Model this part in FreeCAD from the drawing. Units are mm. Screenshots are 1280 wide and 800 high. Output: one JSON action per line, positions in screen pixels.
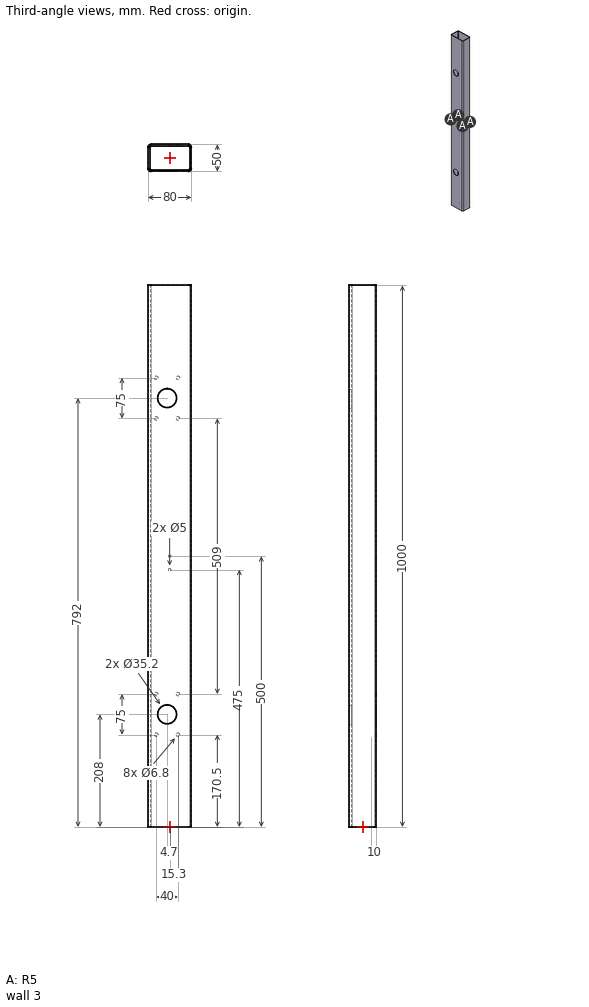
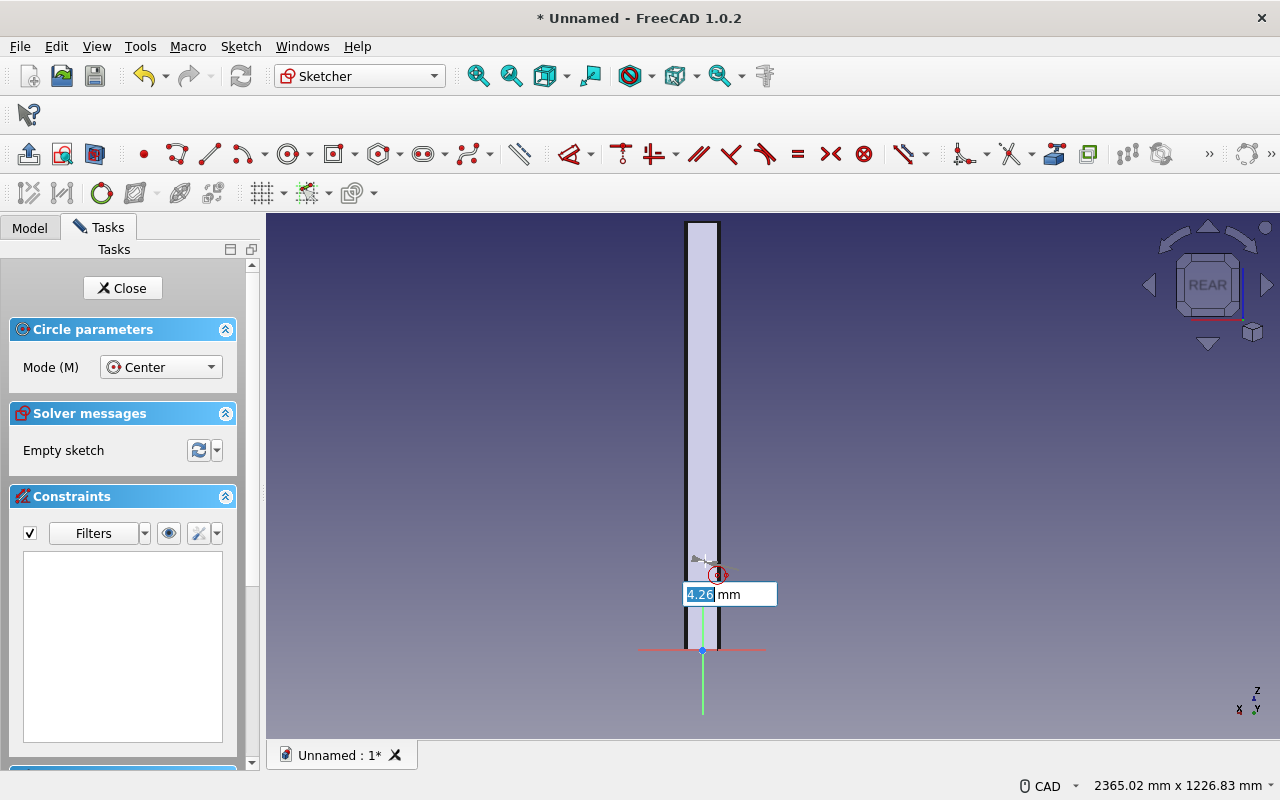
{"action": "scroll", "coordinate": [710, 556], "scroll_direction": "up", "scroll_amount": 4}
{"action": "mouse_move", "coordinate": [709, 555]}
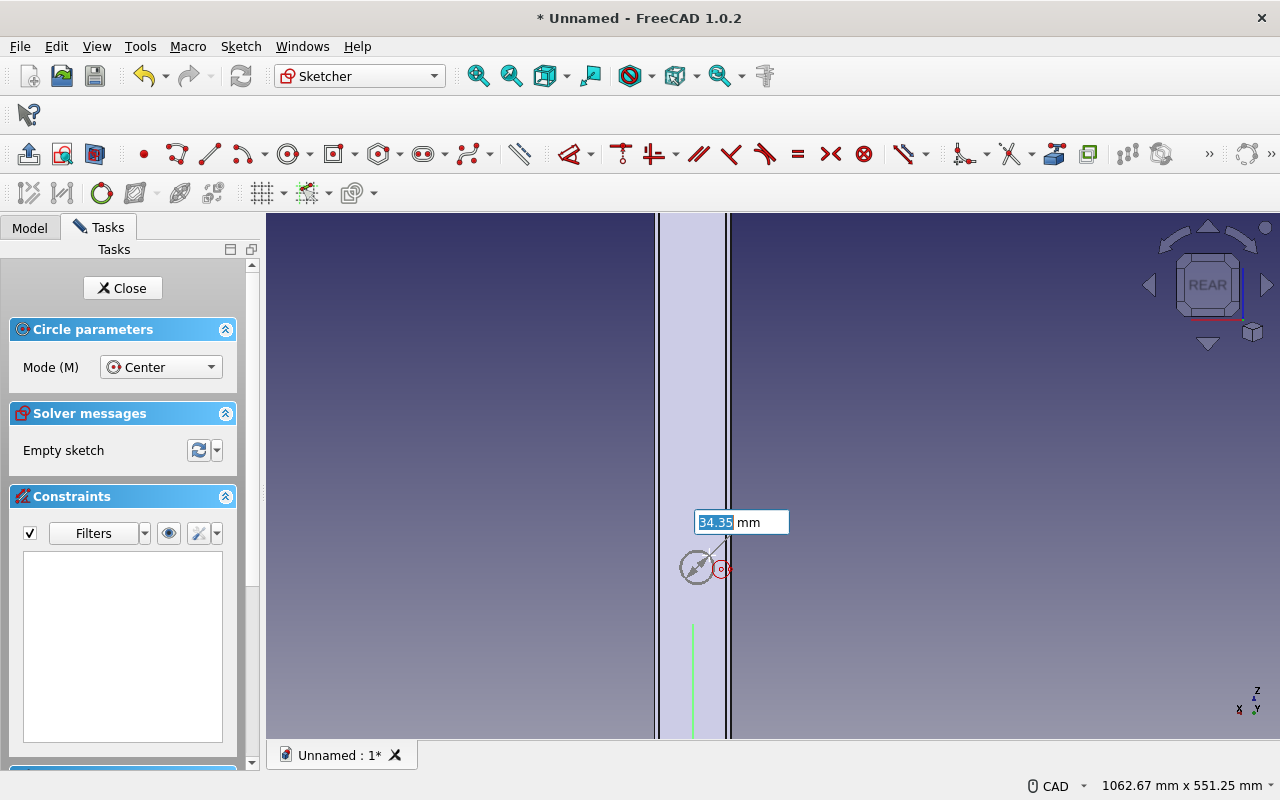
{"action": "type", "text": "35.2"}
{"action": "key", "text": "Return"}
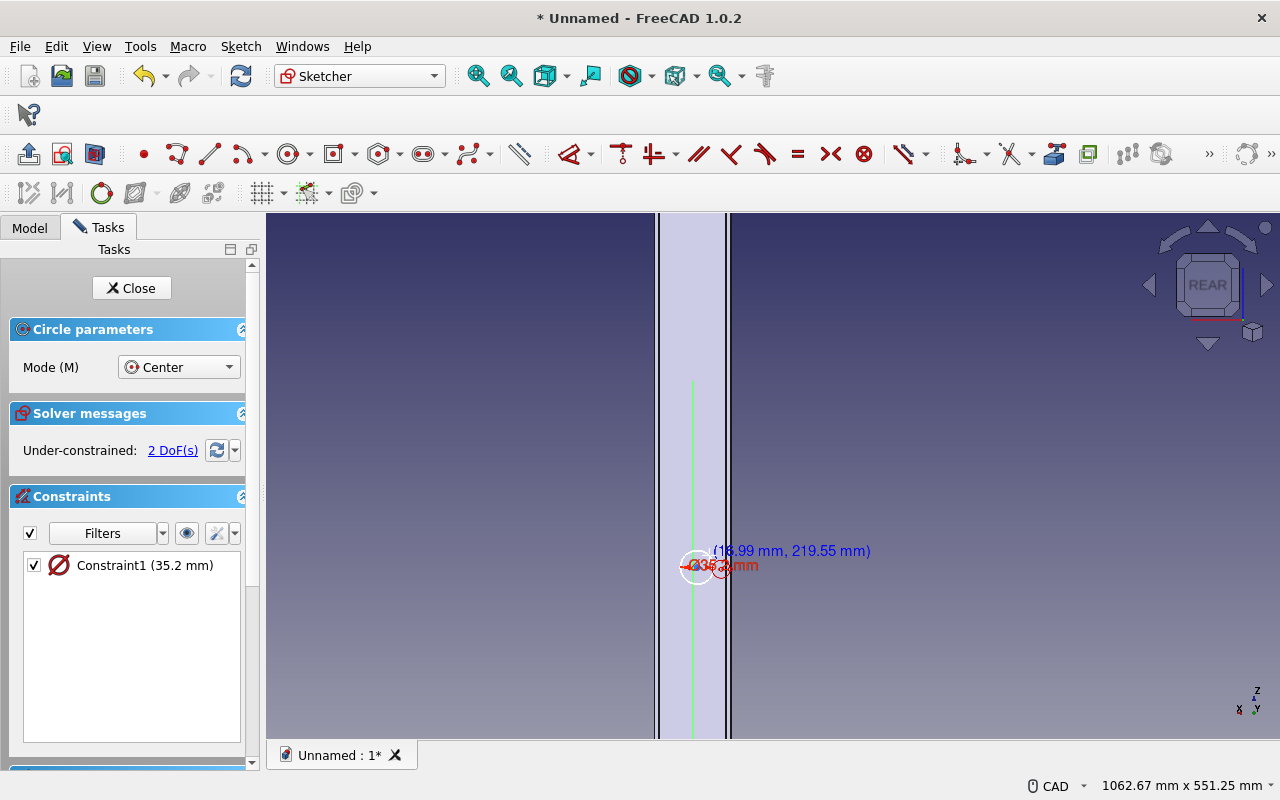
{"action": "scroll", "coordinate": [710, 555], "scroll_direction": "down", "scroll_amount": 4}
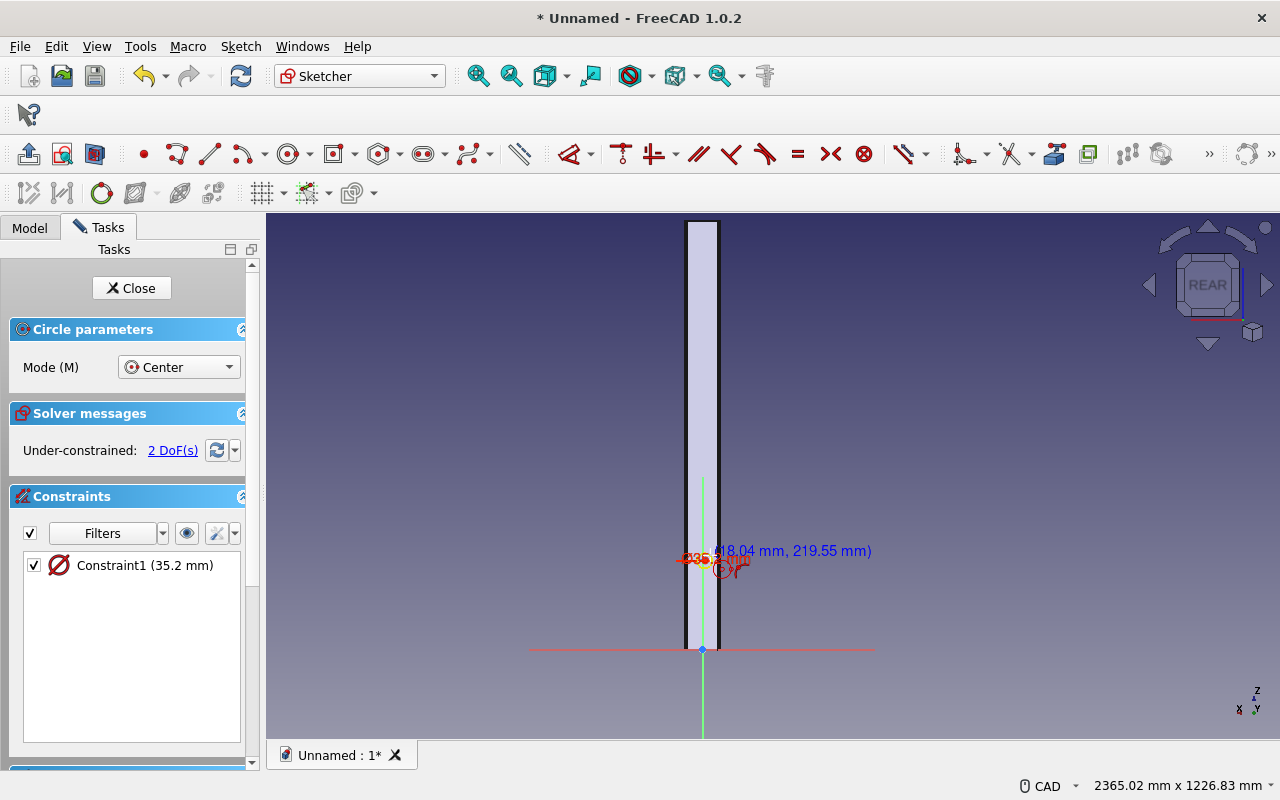
{"action": "scroll", "coordinate": [705, 310], "scroll_direction": "up", "scroll_amount": 11}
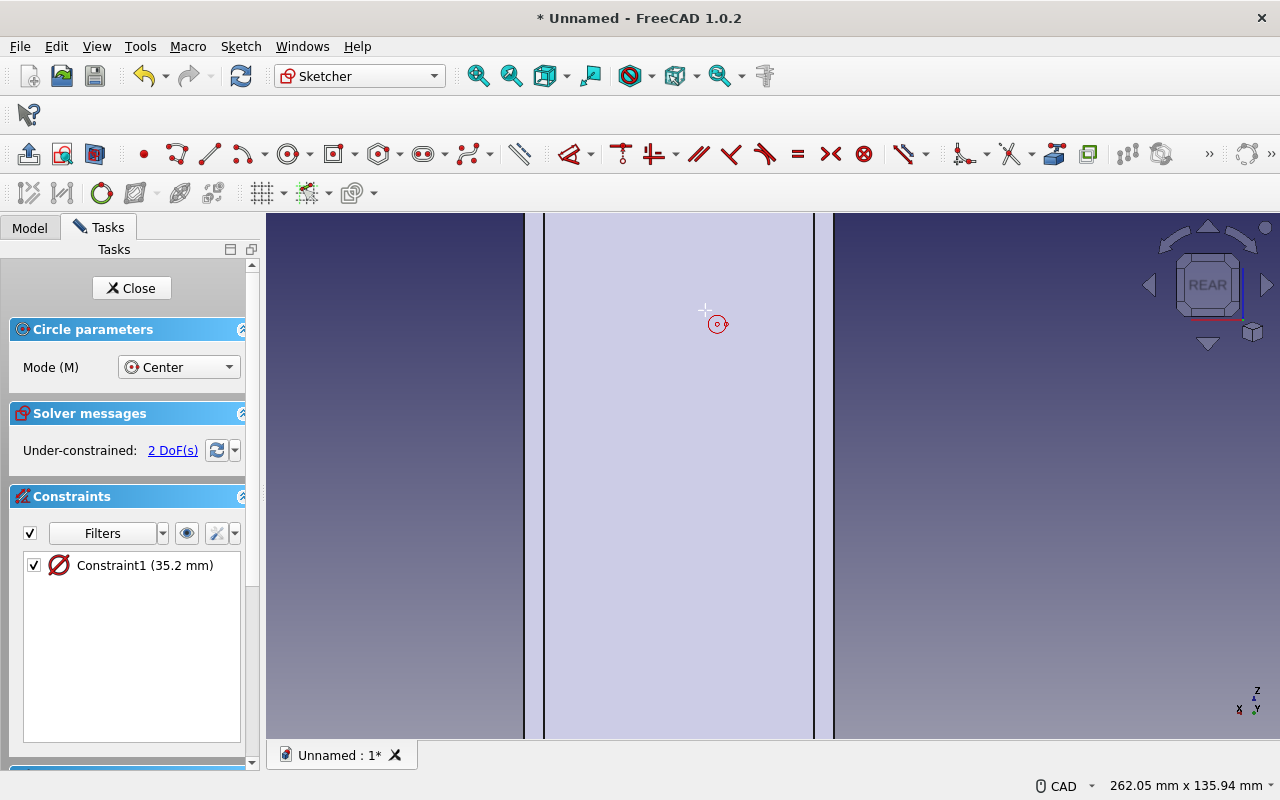
{"action": "left_click", "coordinate": [697, 312]}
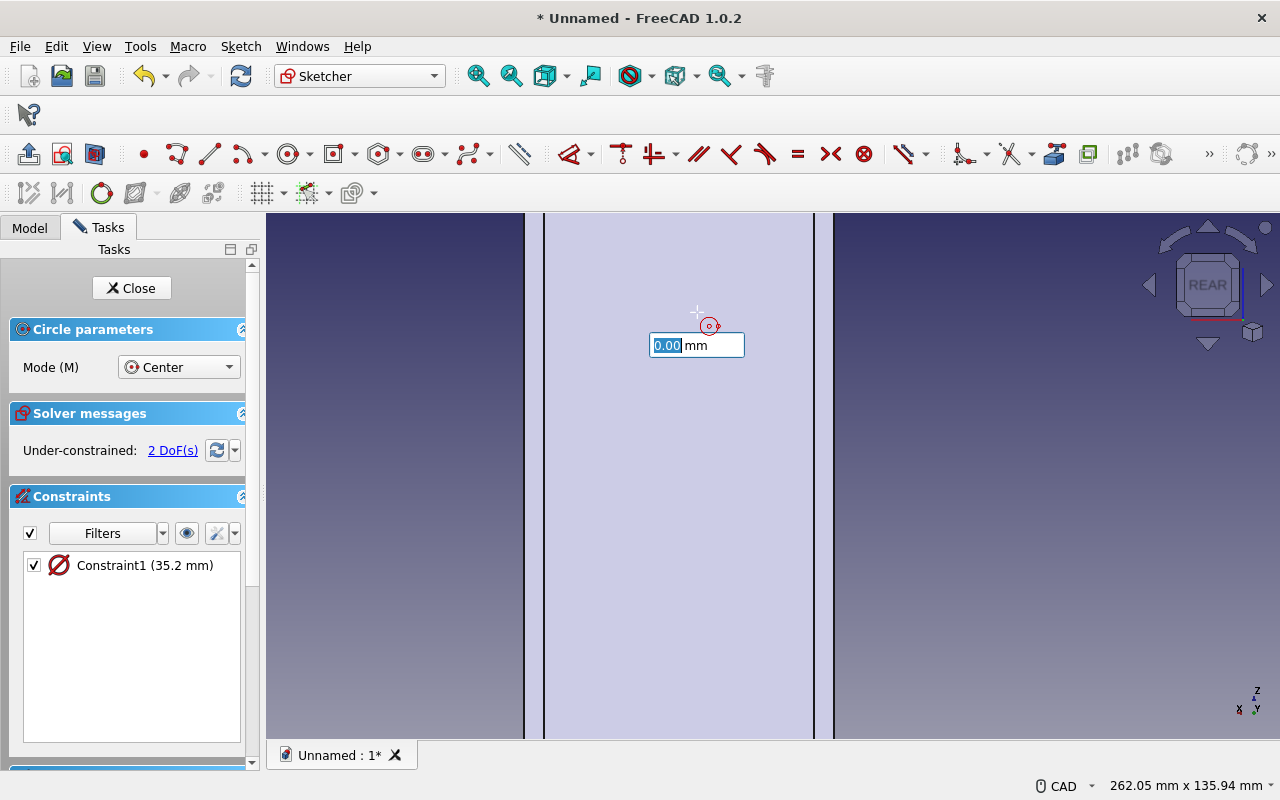
{"action": "scroll", "coordinate": [705, 310], "scroll_direction": "down", "scroll_amount": 11}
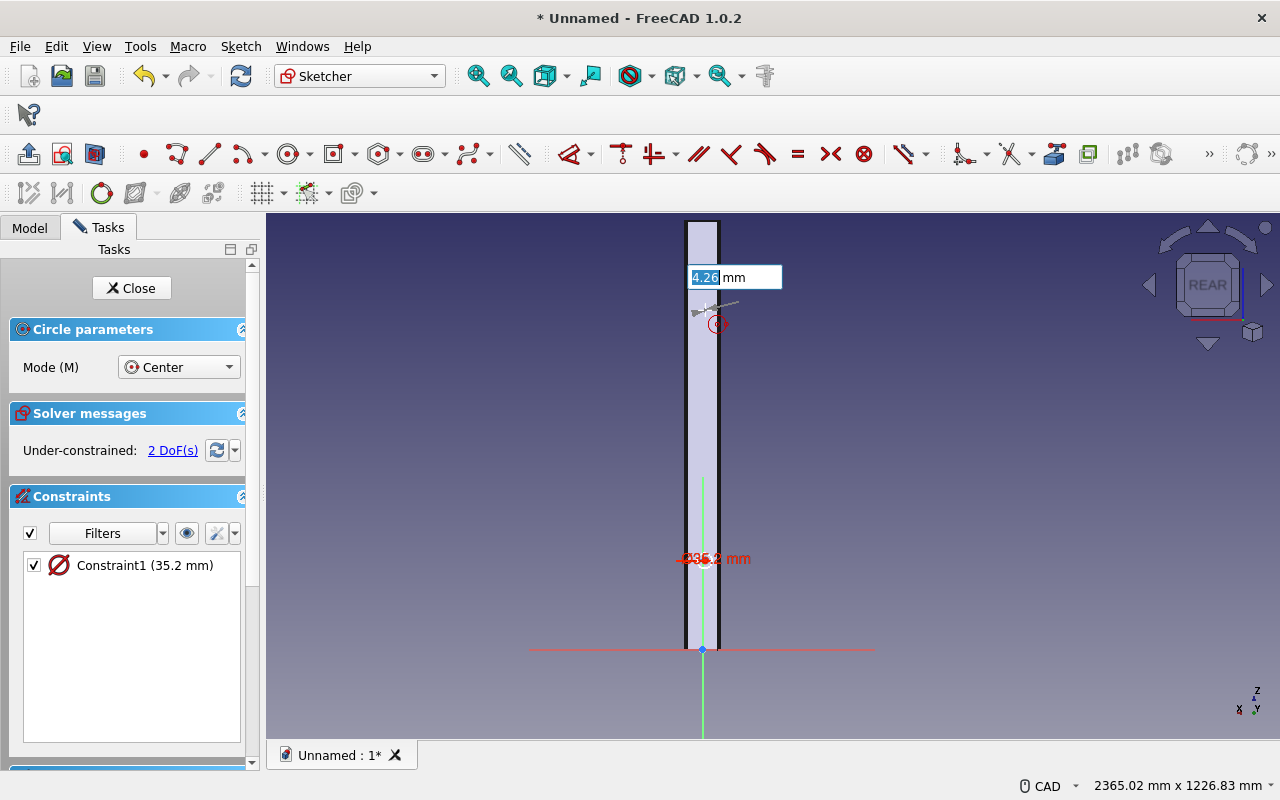
{"action": "scroll", "coordinate": [710, 305], "scroll_direction": "up", "scroll_amount": 4}
{"action": "mouse_move", "coordinate": [709, 305]}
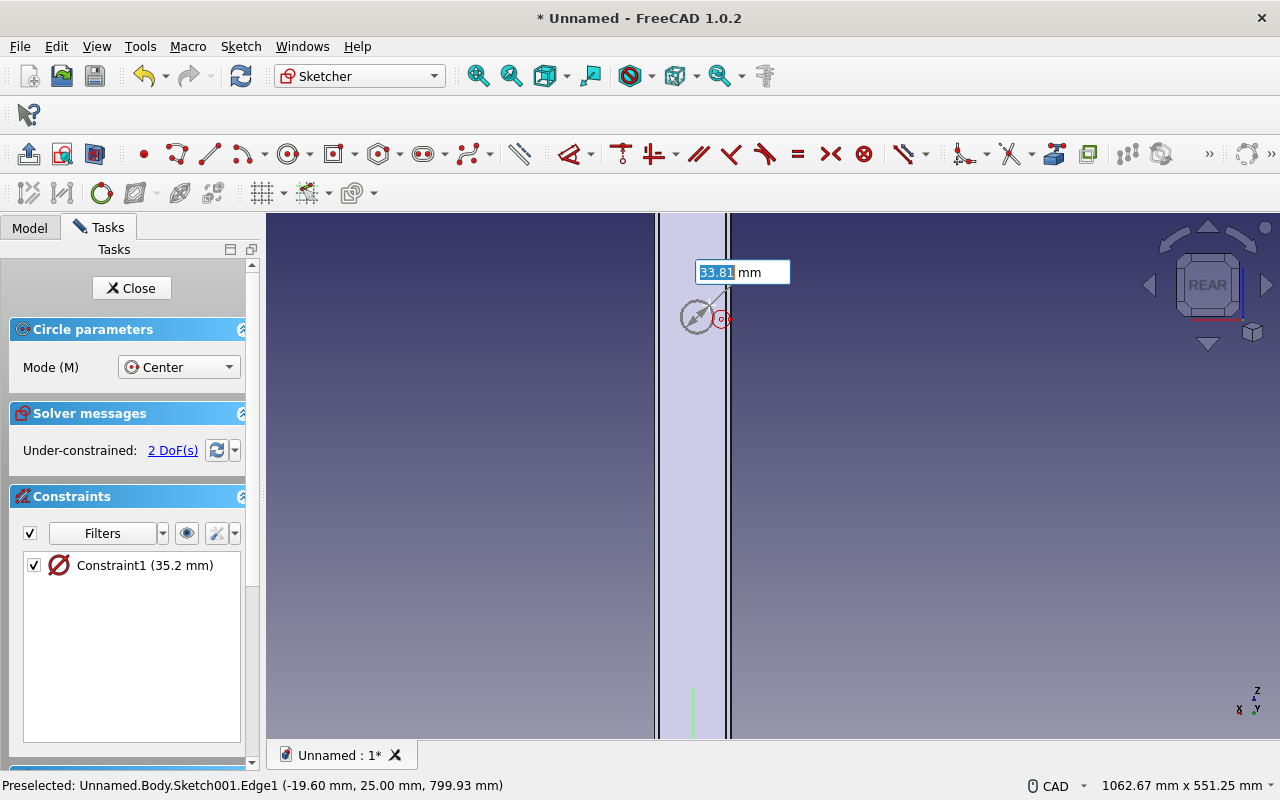
{"action": "type", "text": "35.2"}
{"action": "key", "text": "Return"}
{"action": "key", "text": "Escape"}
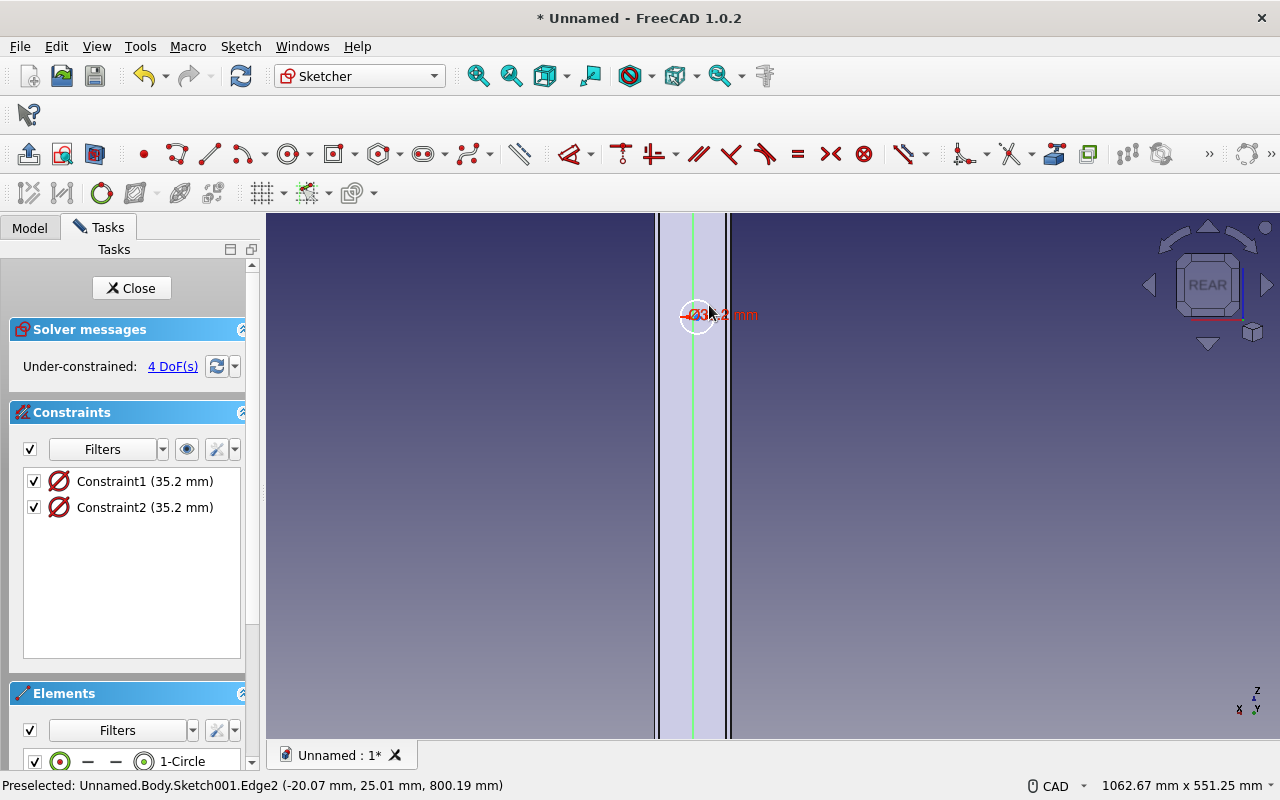
{"action": "scroll", "coordinate": [710, 304], "scroll_direction": "down", "scroll_amount": 4}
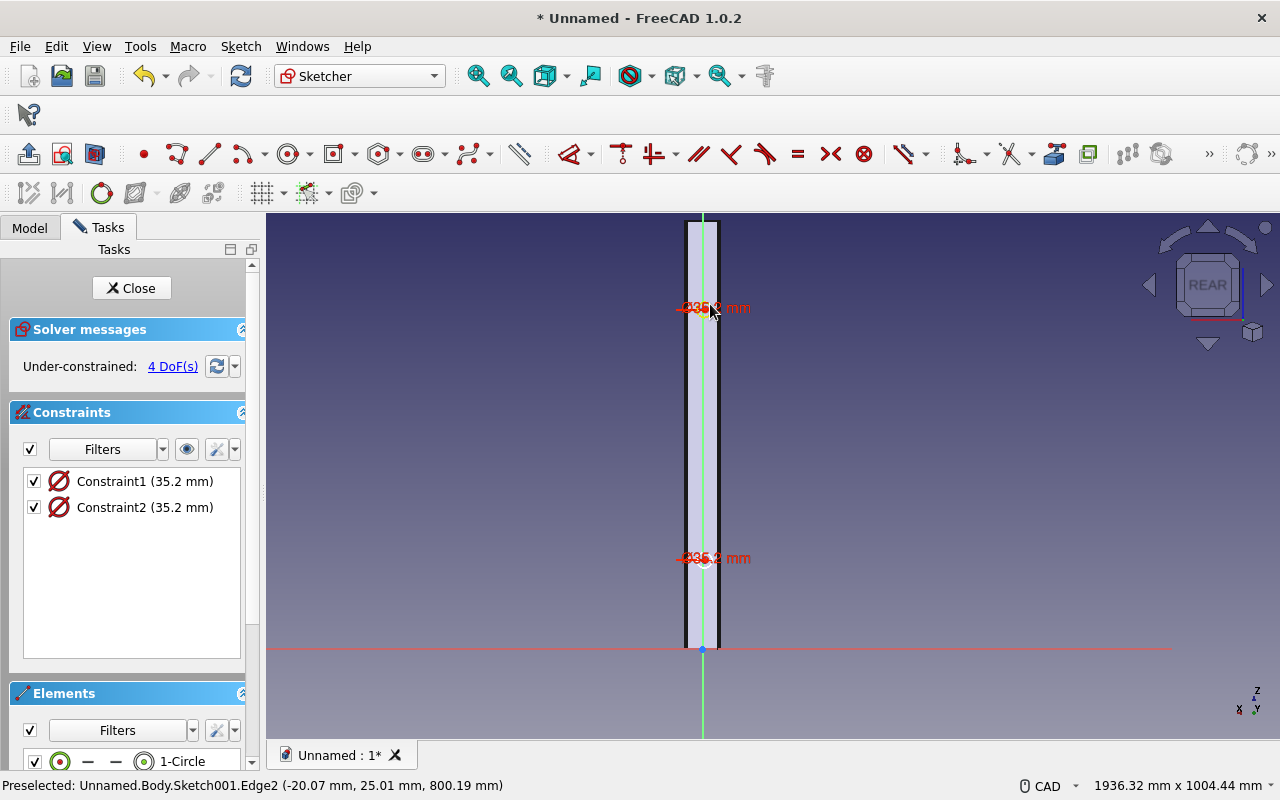
{"action": "scroll", "coordinate": [704, 560], "scroll_direction": "up", "scroll_amount": 15}